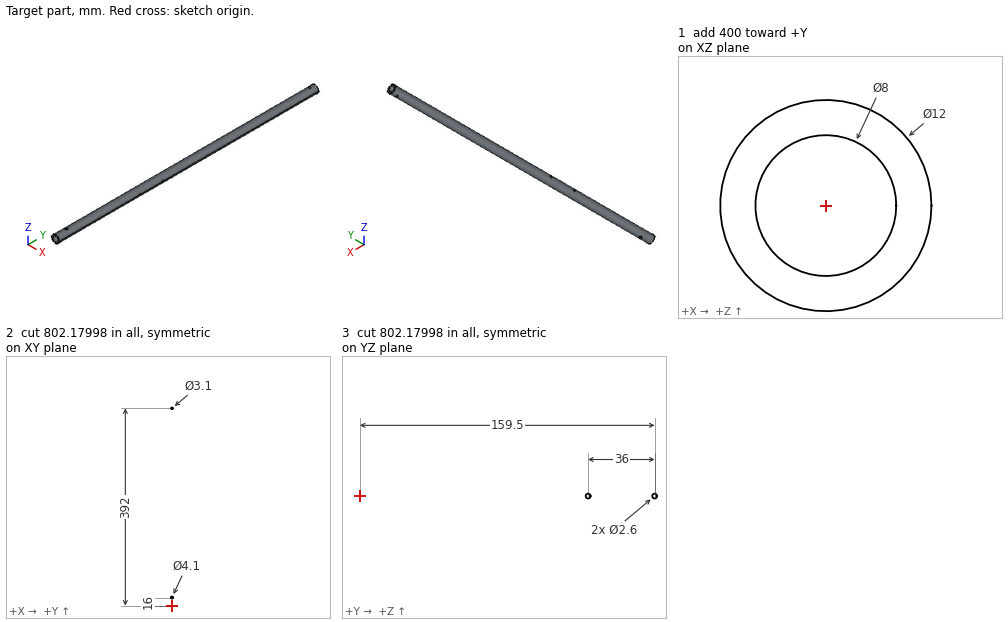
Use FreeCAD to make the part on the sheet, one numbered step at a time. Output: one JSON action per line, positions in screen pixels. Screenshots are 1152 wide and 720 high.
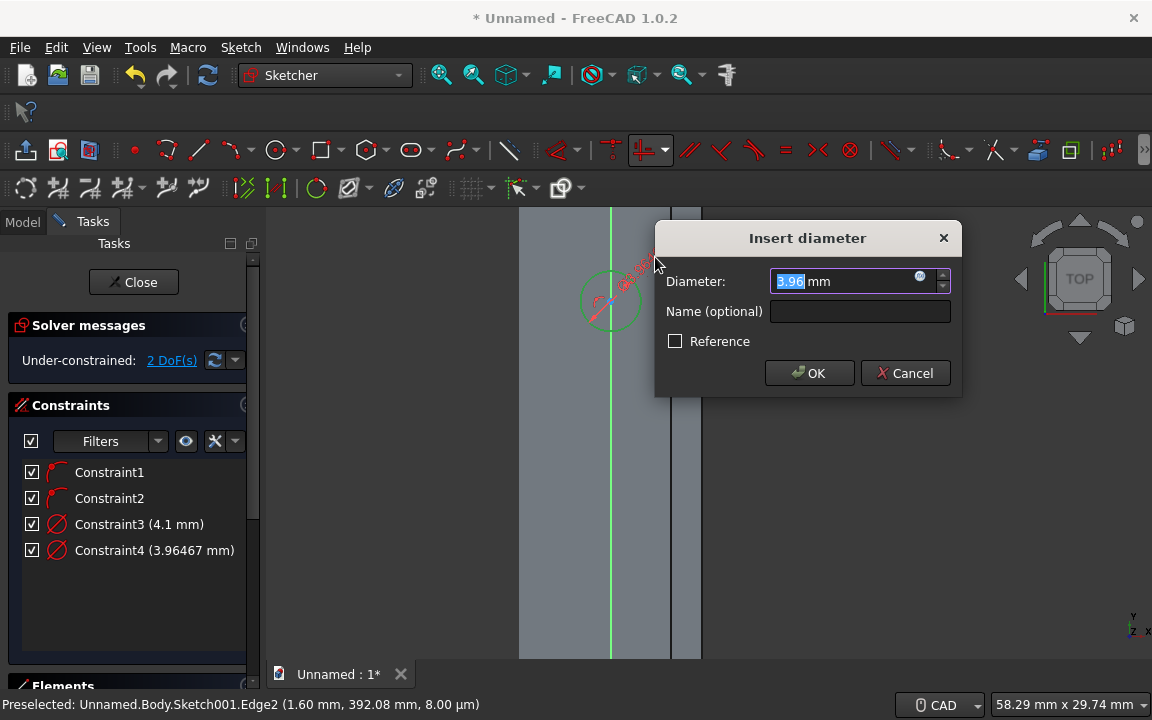
{"action": "type", "text": "3.1"}
{"action": "key", "text": "Return"}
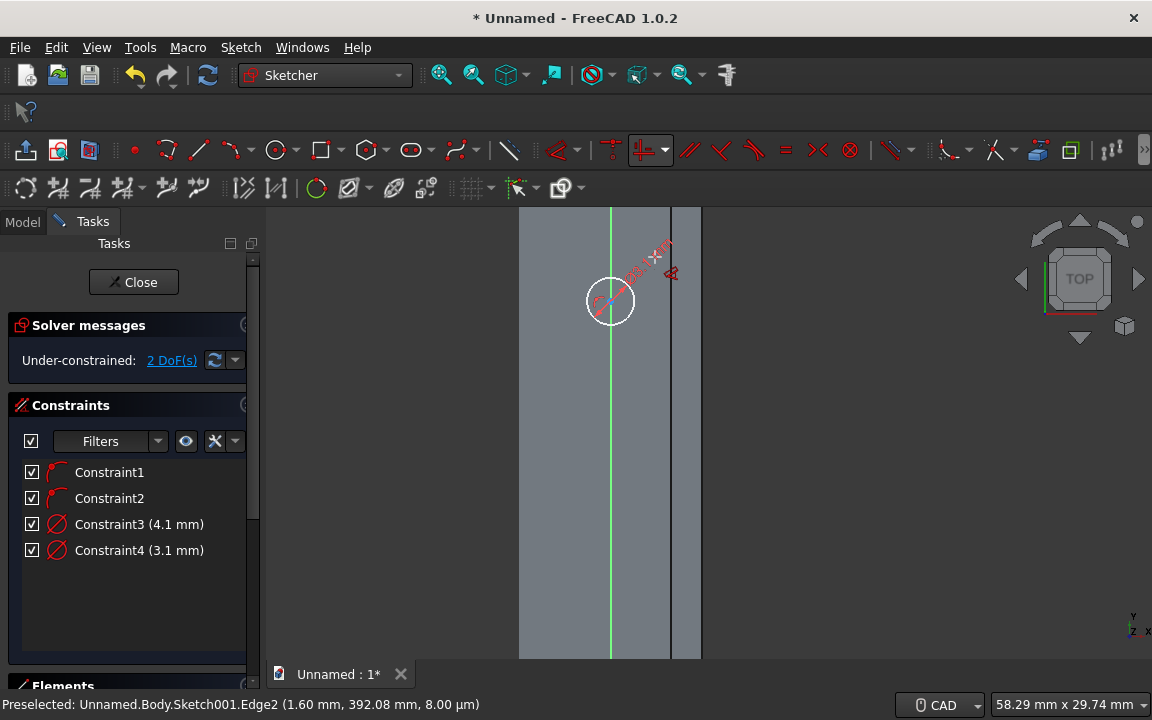
{"action": "scroll", "coordinate": [642, 285], "scroll_direction": "down", "scroll_amount": 15}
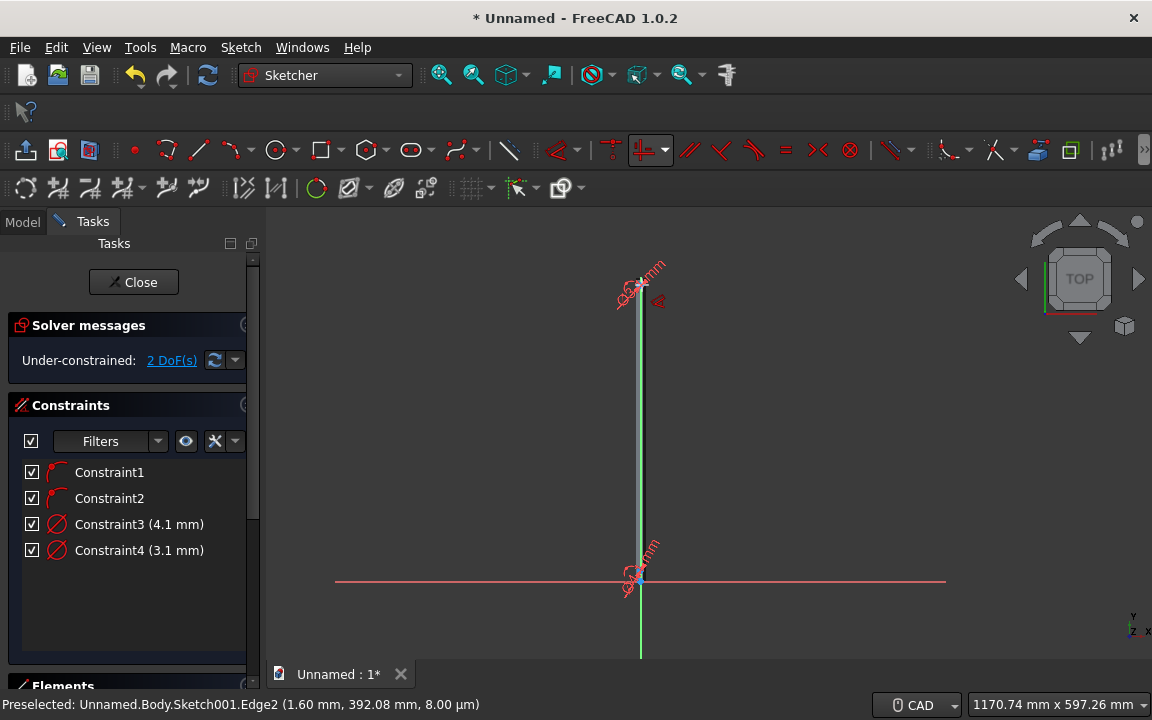
{"action": "scroll", "coordinate": [641, 571], "scroll_direction": "up", "scroll_amount": 6}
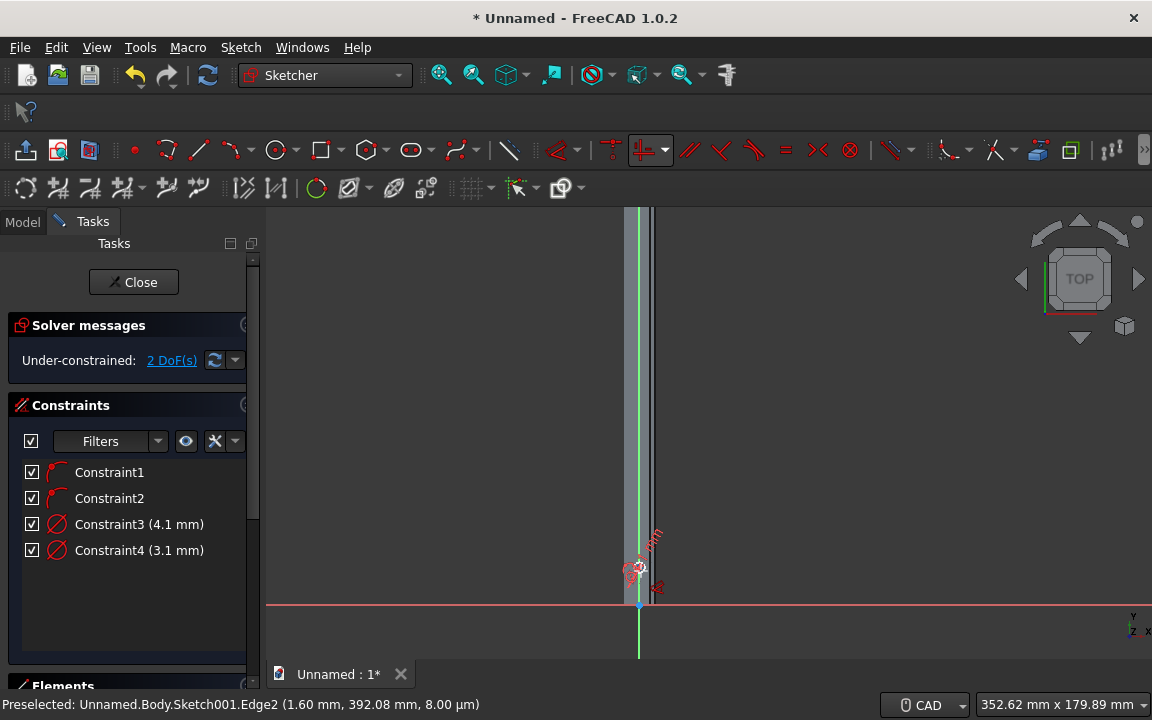
{"action": "left_click", "coordinate": [639, 568]}
{"action": "left_click", "coordinate": [673, 586]}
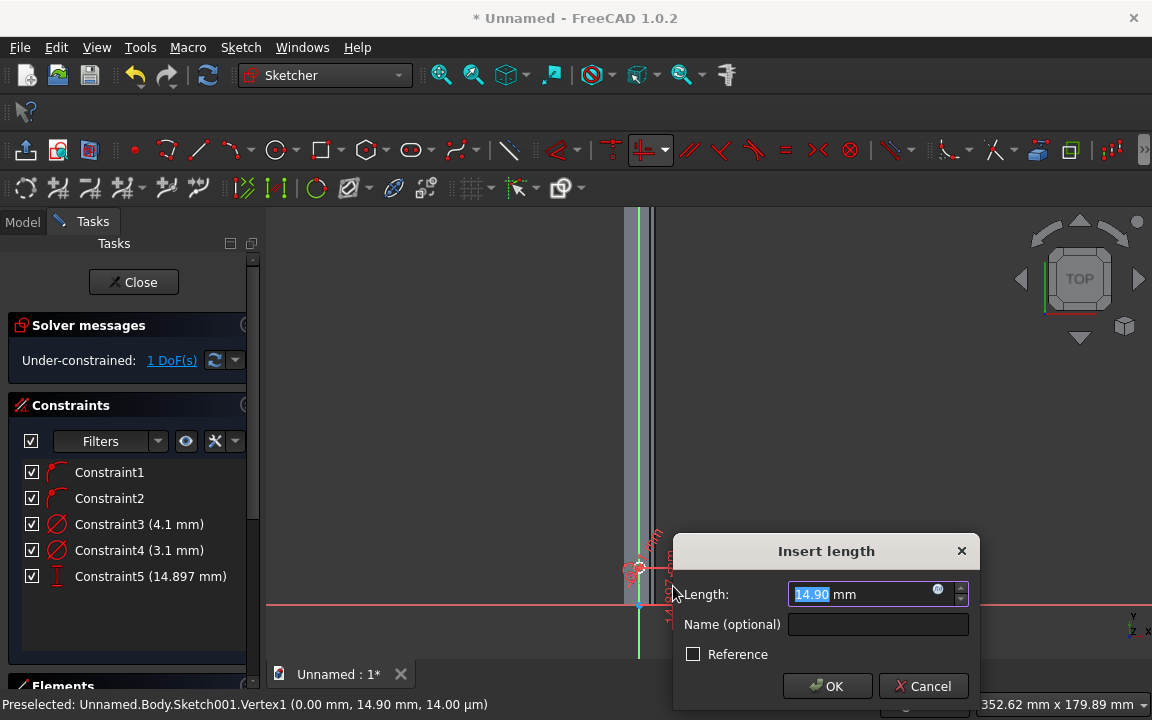
{"action": "type", "text": "16"}
{"action": "key", "text": "Return"}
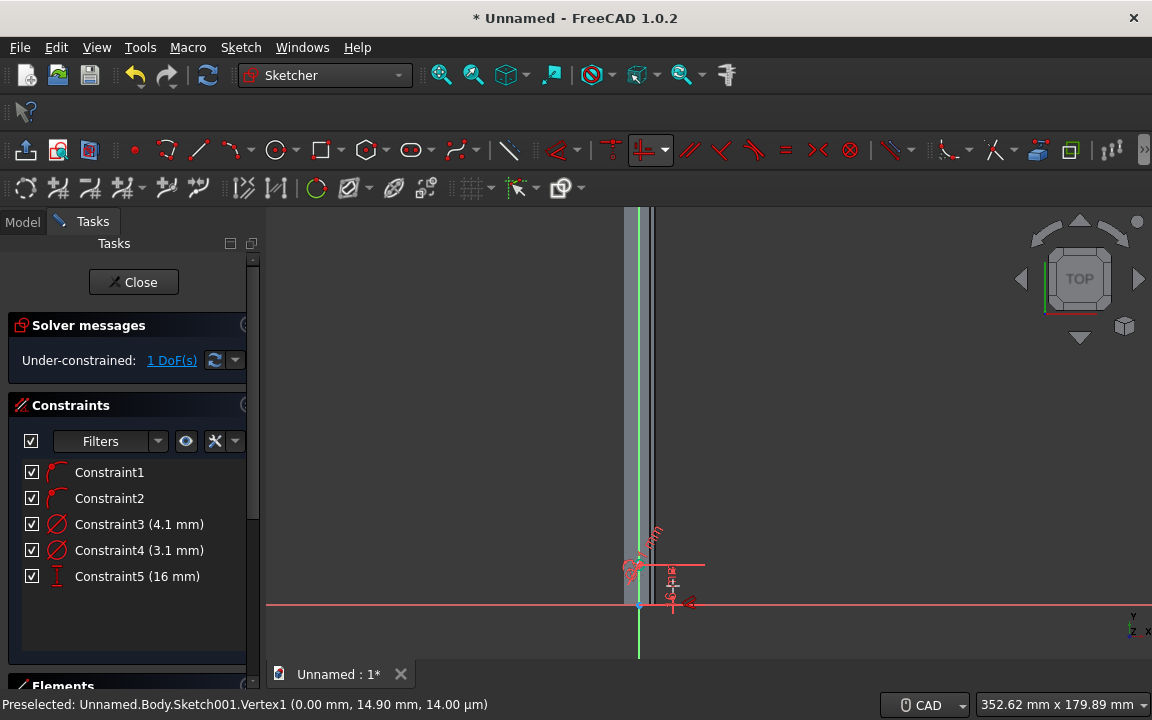
{"action": "scroll", "coordinate": [641, 572], "scroll_direction": "down", "scroll_amount": 6}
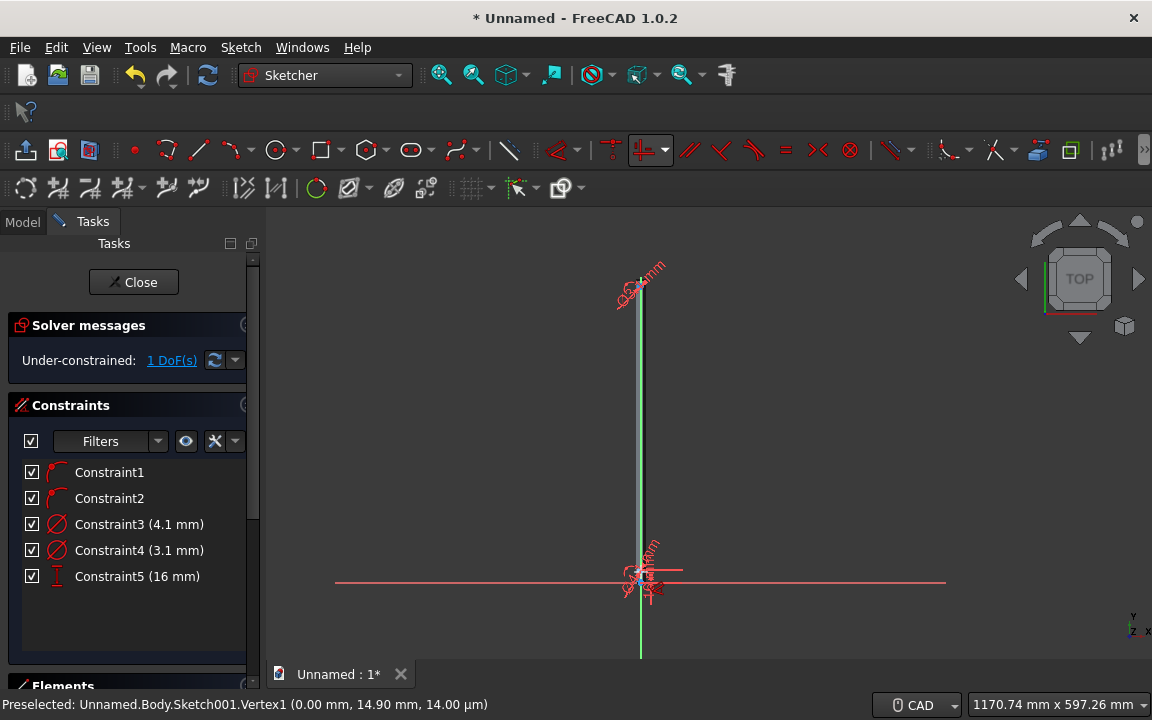
{"action": "left_click", "coordinate": [641, 287]}
{"action": "left_click", "coordinate": [675, 435]}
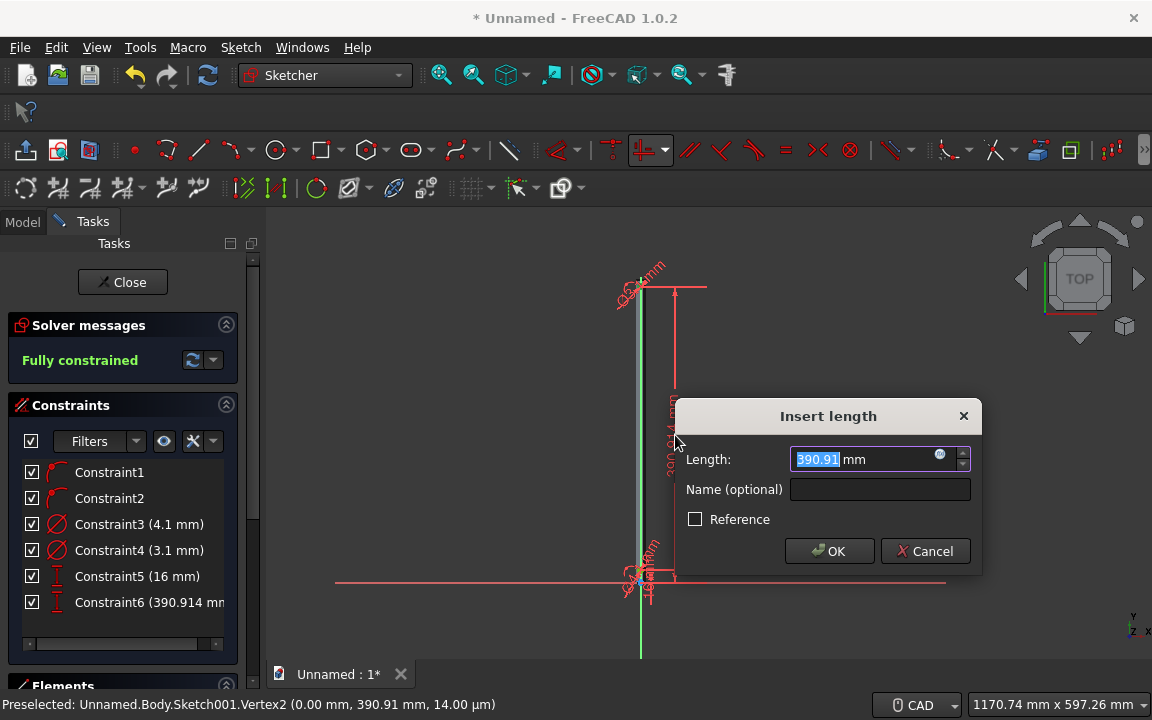
{"action": "type", "text": "392"}
{"action": "key", "text": "Return"}
{"action": "key", "text": "Escape"}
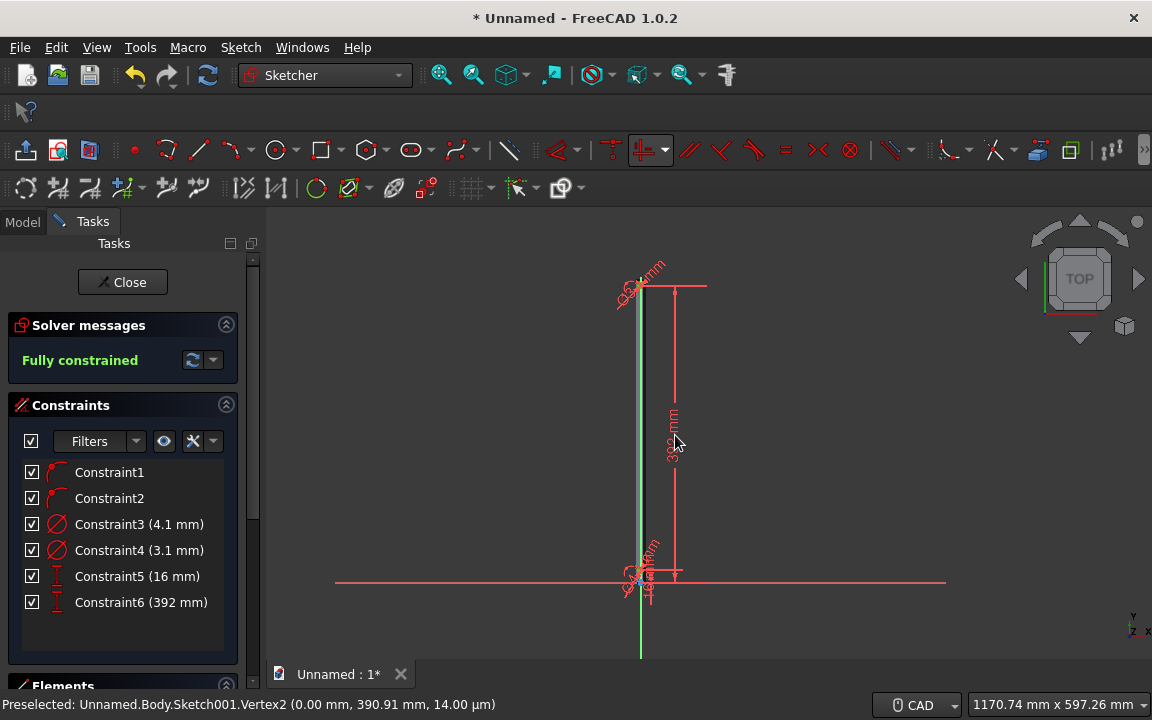
{"action": "left_click", "coordinate": [123, 282]}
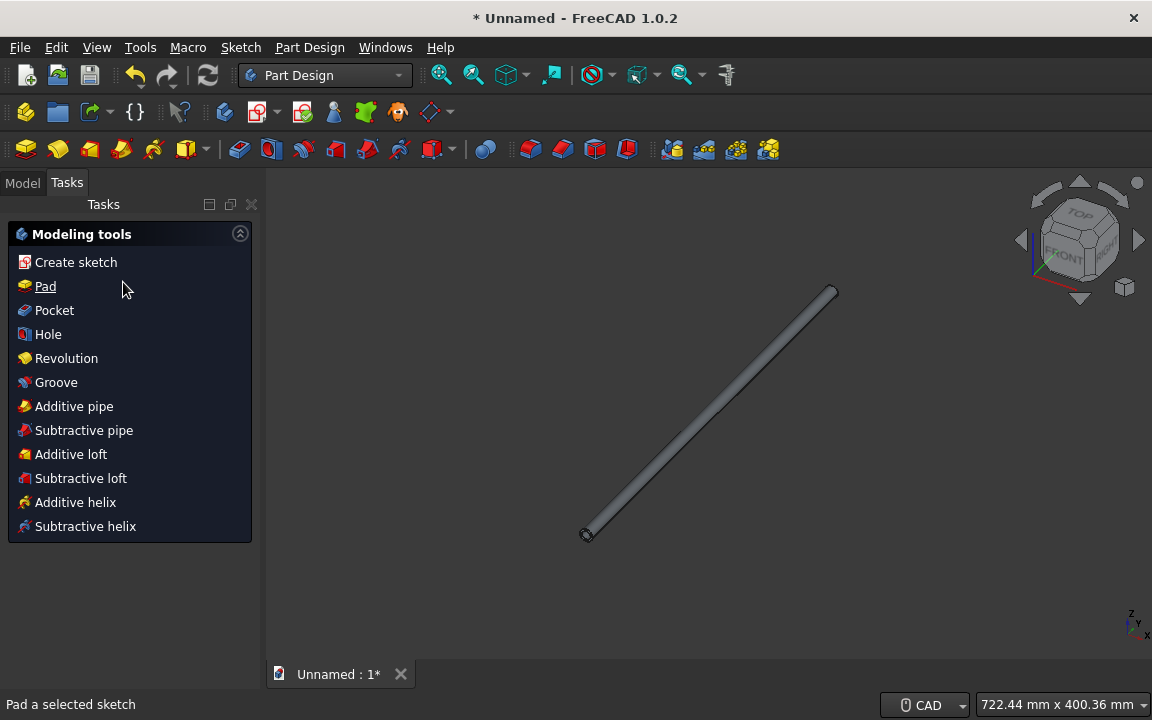
{"action": "left_click", "coordinate": [240, 150]}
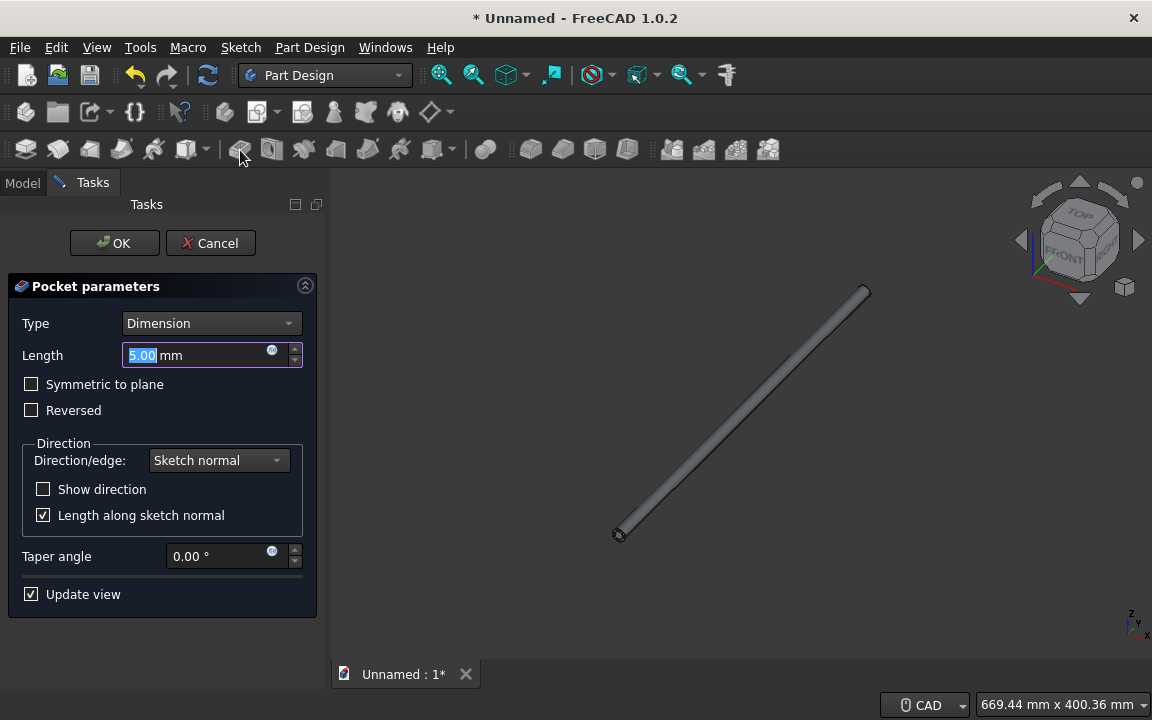
{"action": "type", "text": "802.17998"}
{"action": "key", "text": "Tab"}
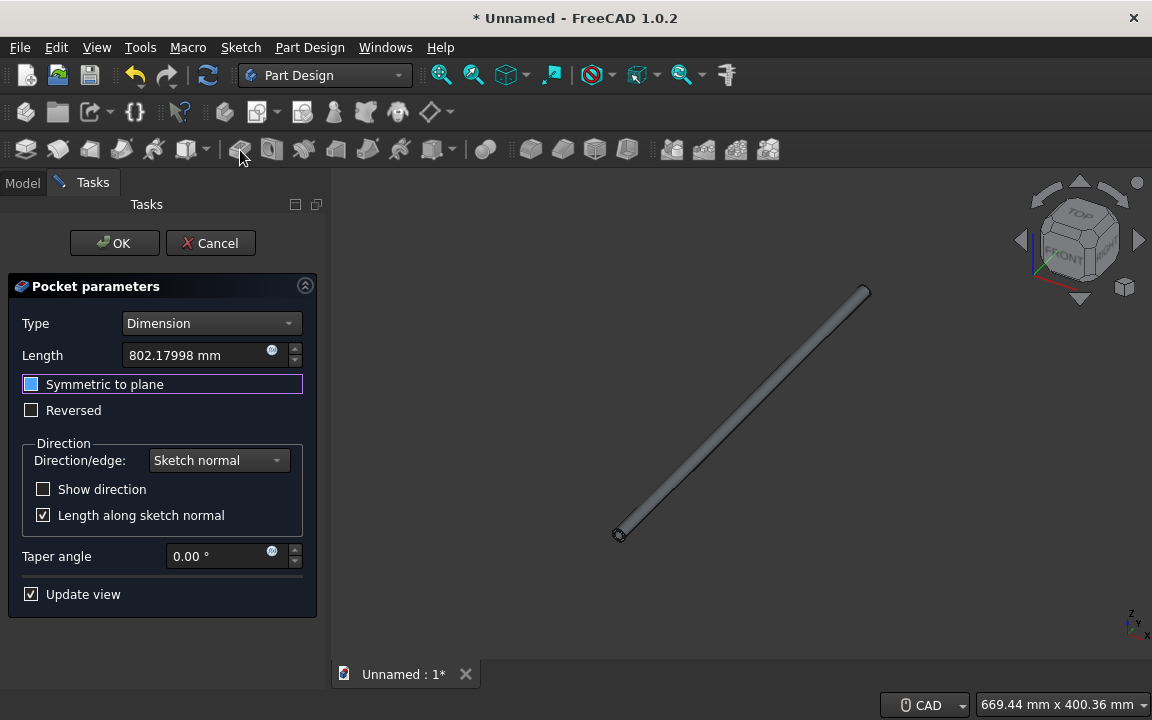
{"action": "left_click", "coordinate": [30, 384]}